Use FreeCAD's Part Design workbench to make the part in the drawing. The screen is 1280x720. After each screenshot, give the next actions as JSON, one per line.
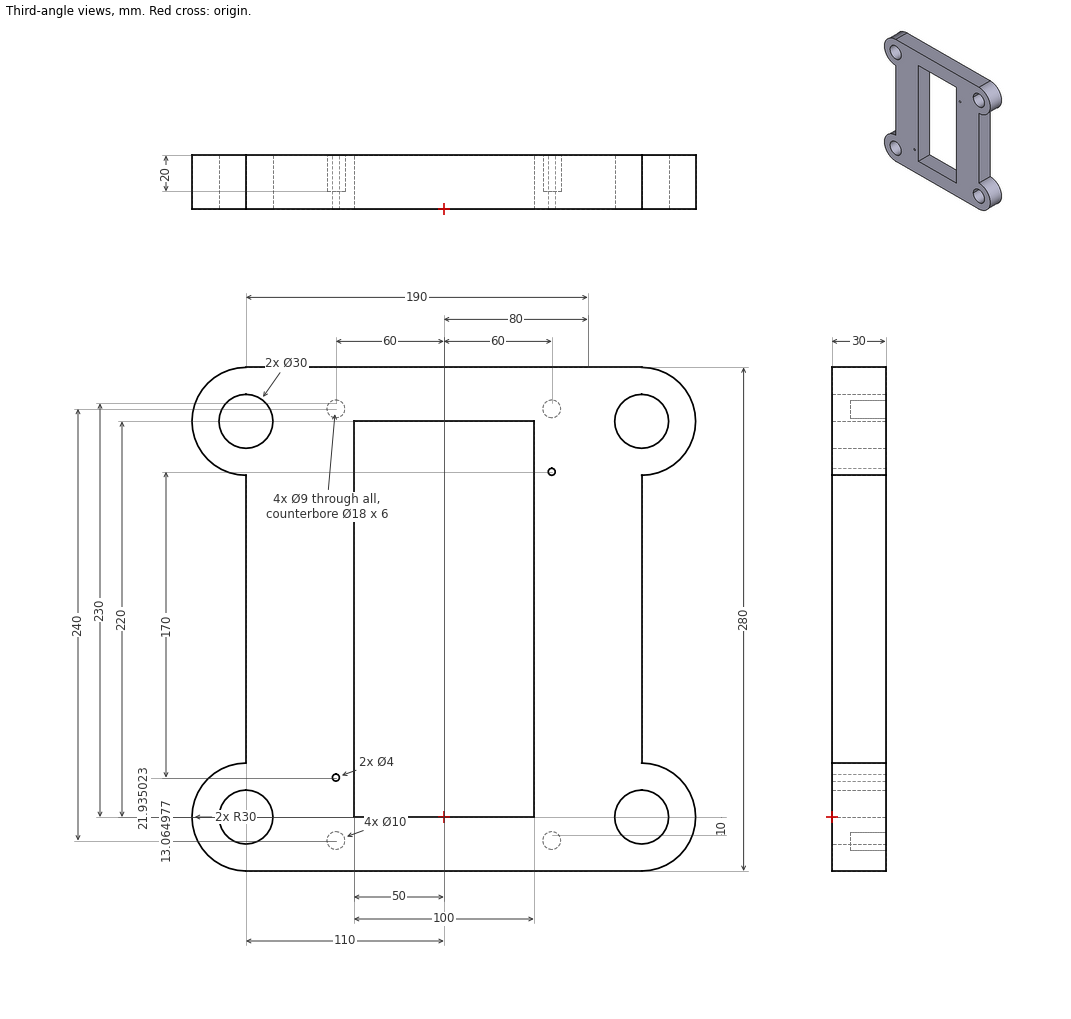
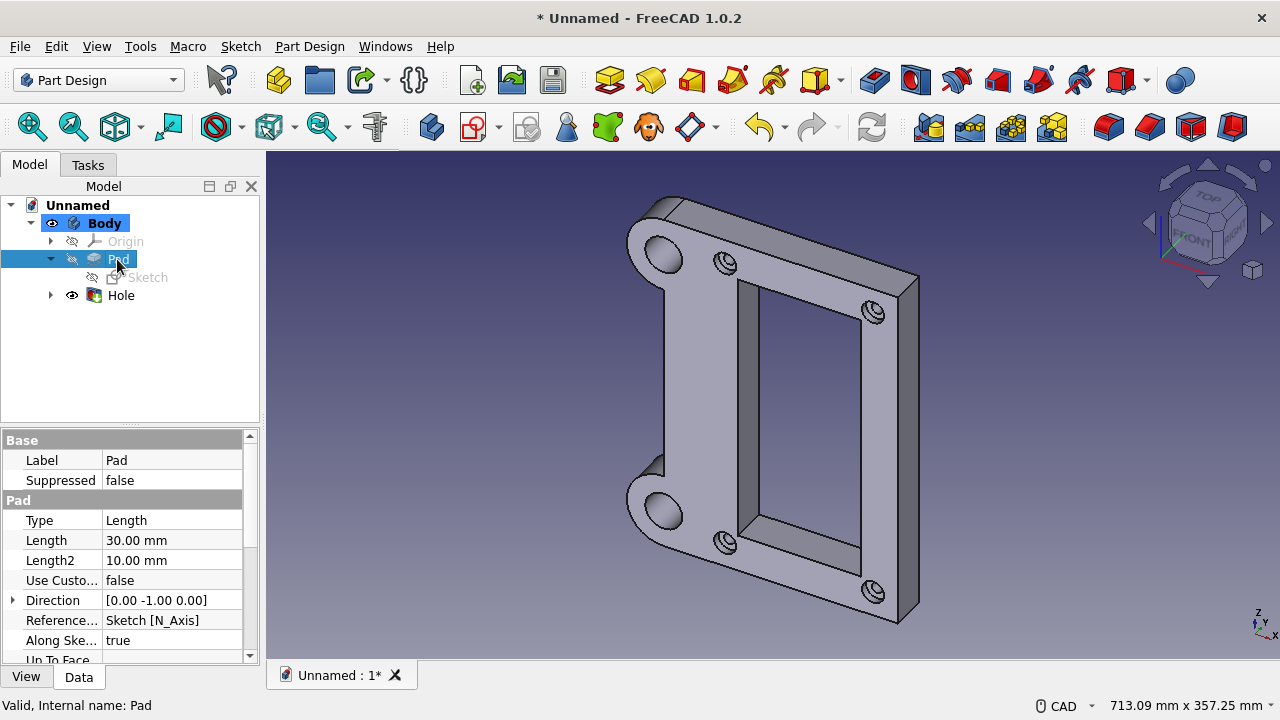
{"action": "left_click", "coordinate": [929, 128]}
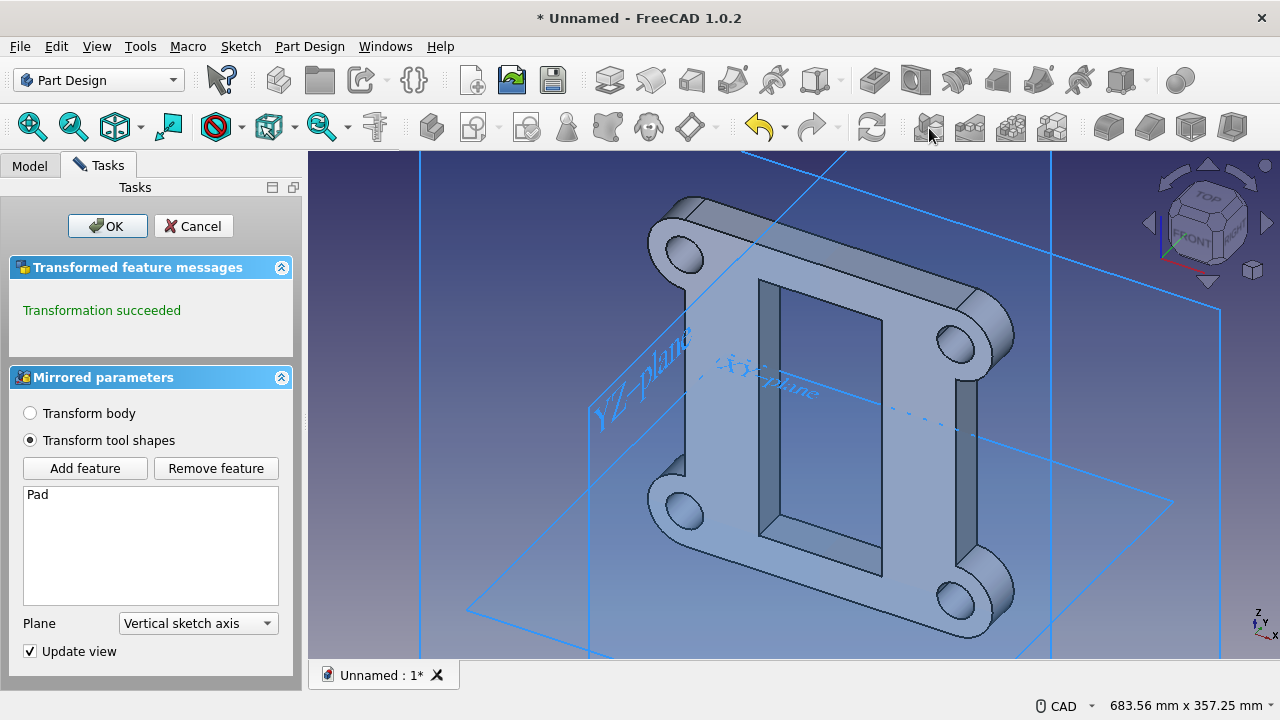
{"action": "left_click", "coordinate": [199, 624]}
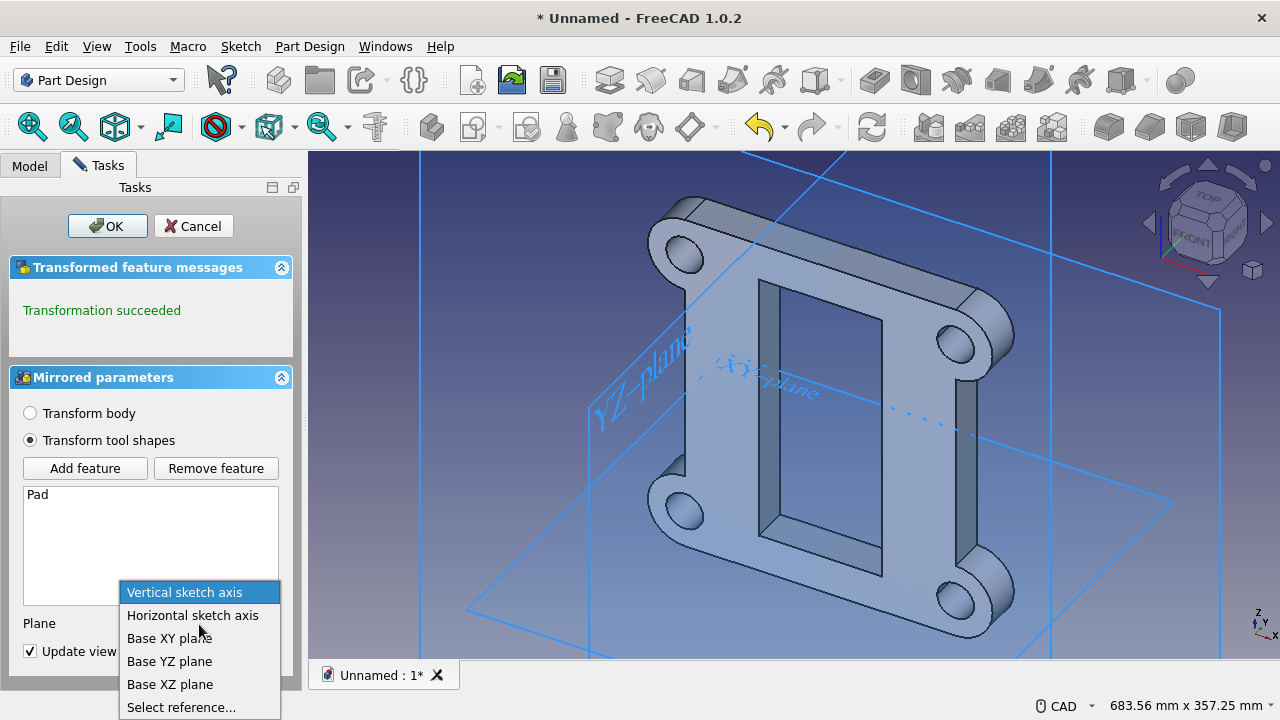
{"action": "left_click", "coordinate": [198, 662]}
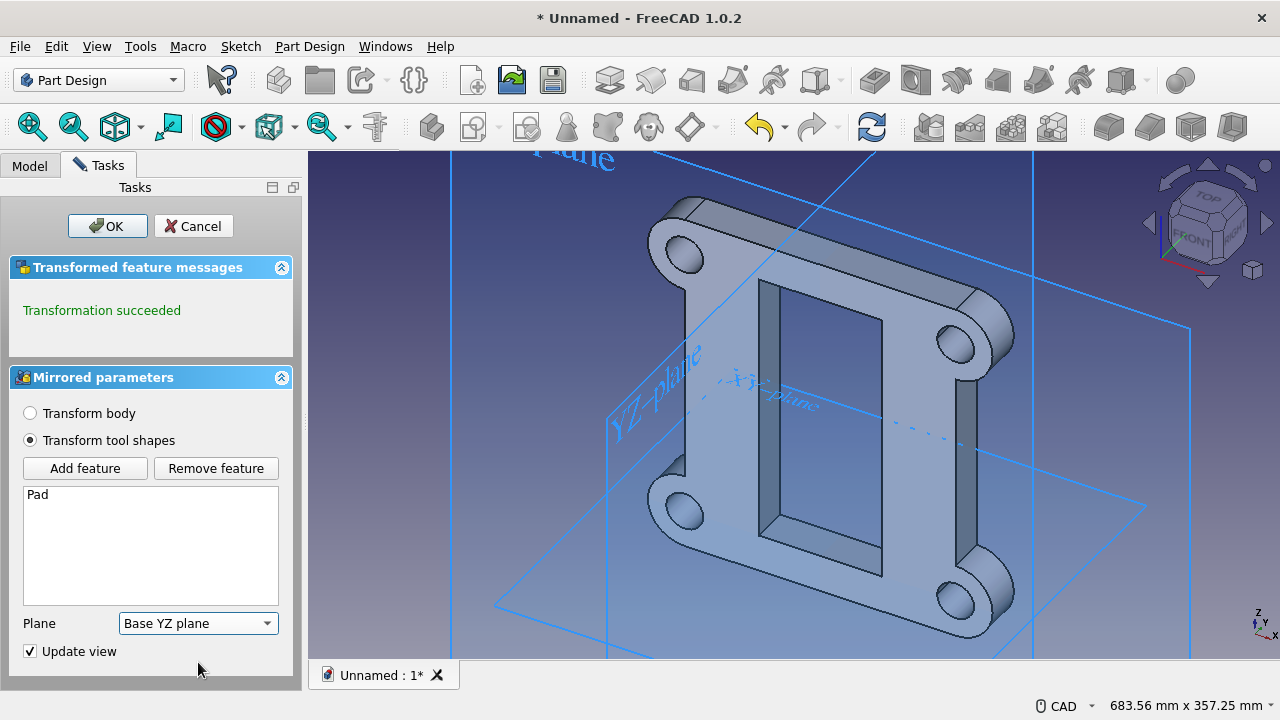
{"action": "left_click", "coordinate": [108, 226]}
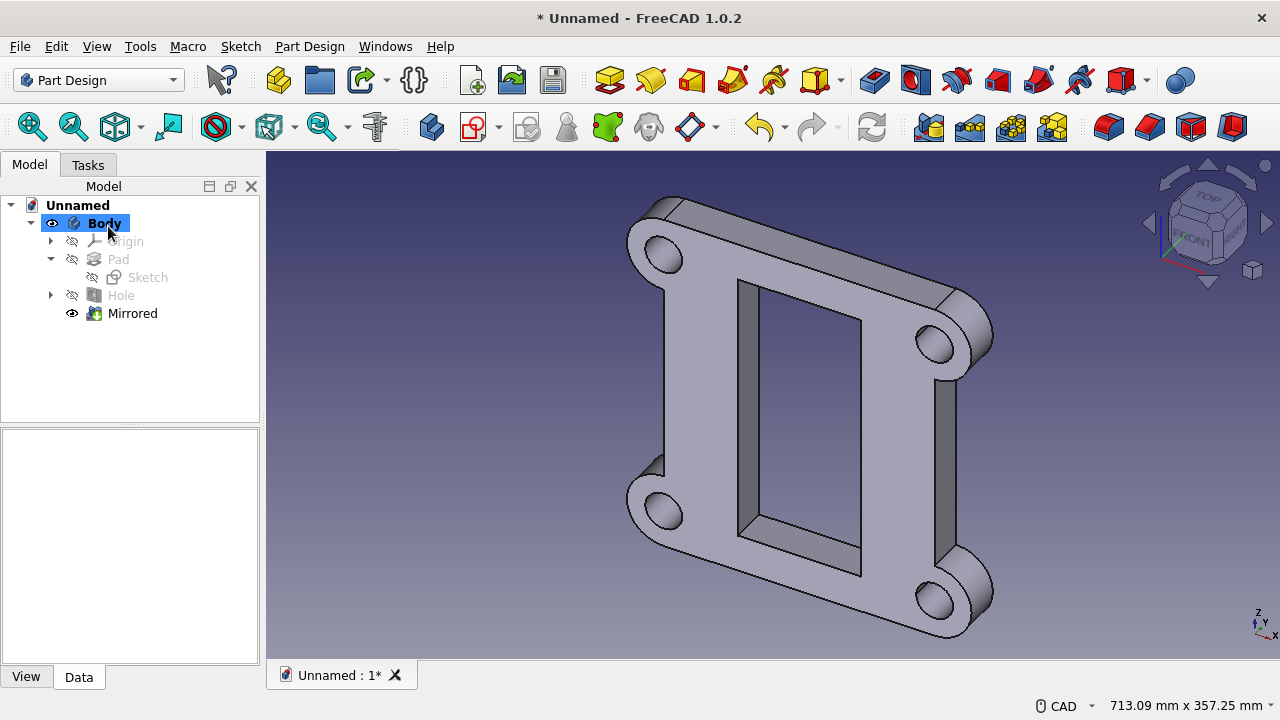
{"action": "key", "text": "4"}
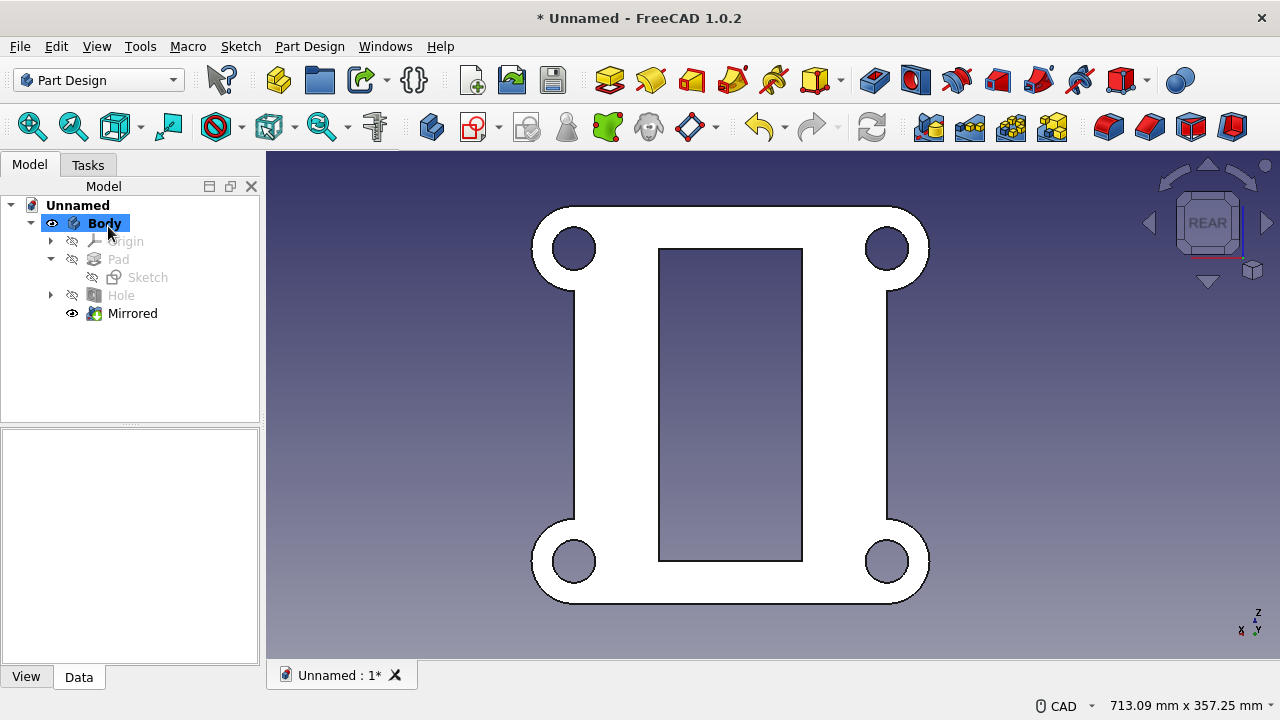
{"action": "left_click", "coordinate": [844, 347]}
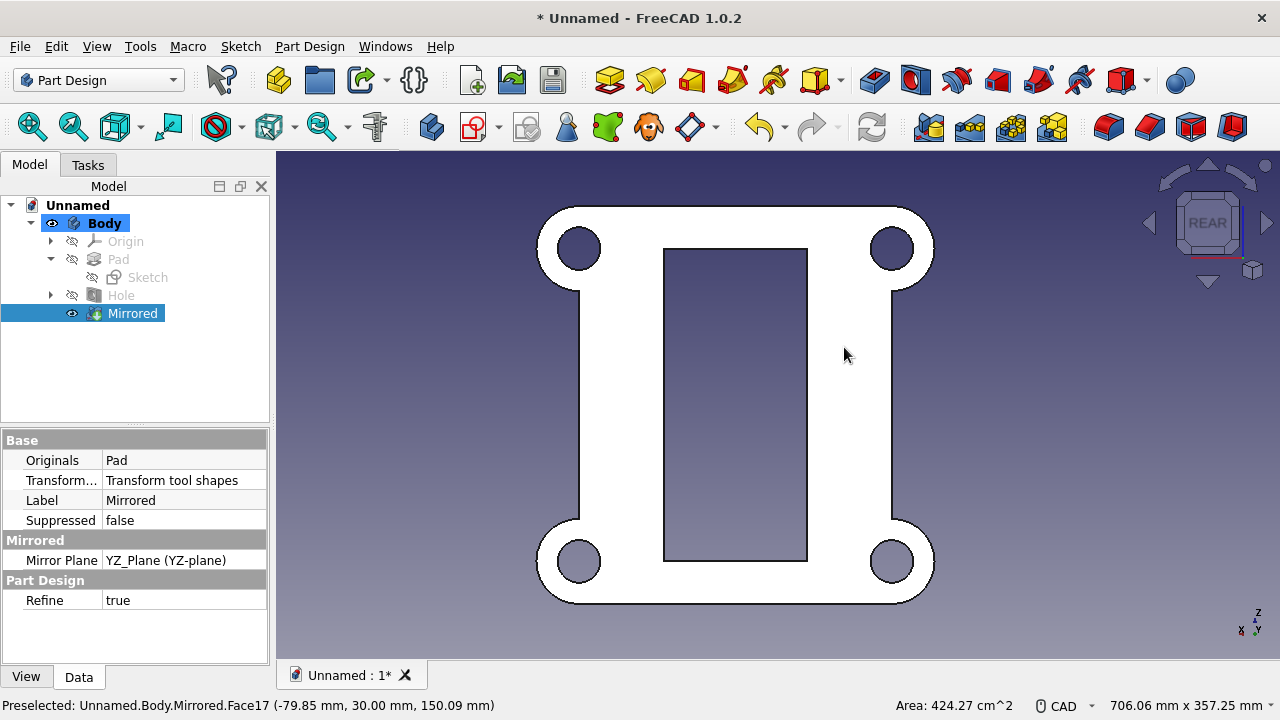
{"action": "left_click", "coordinate": [472, 128]}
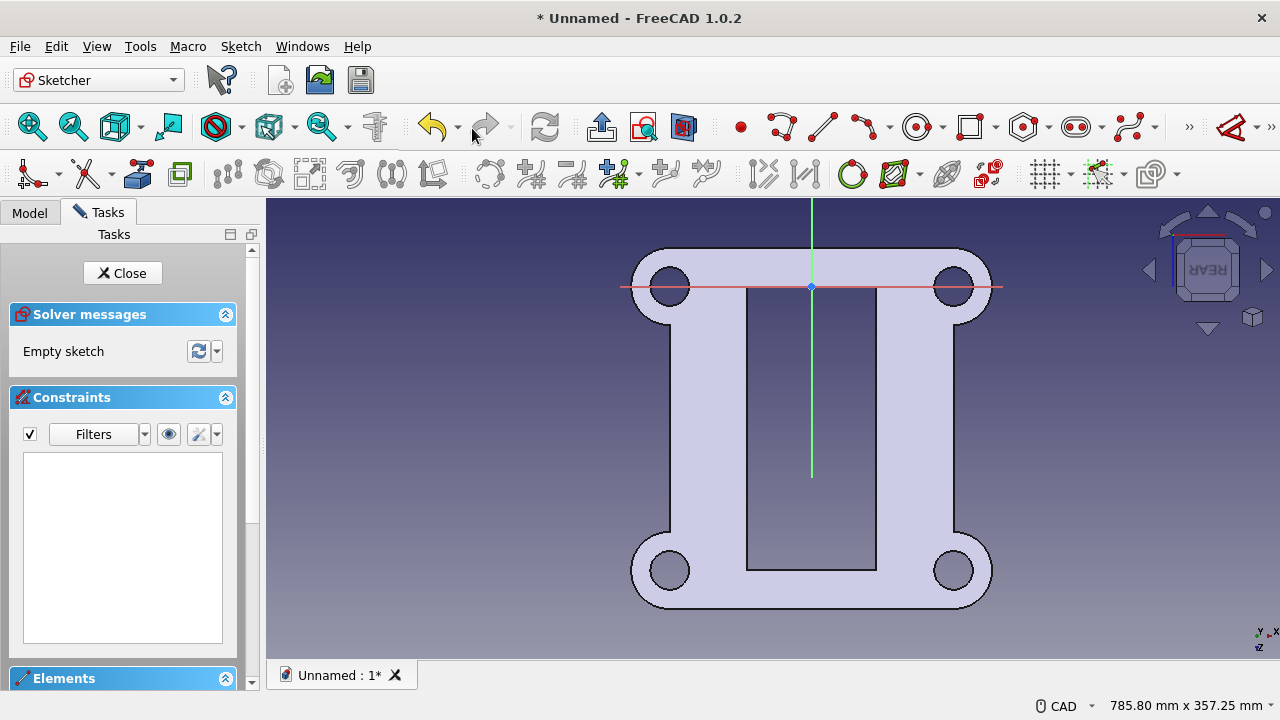
{"action": "key", "text": "g c"}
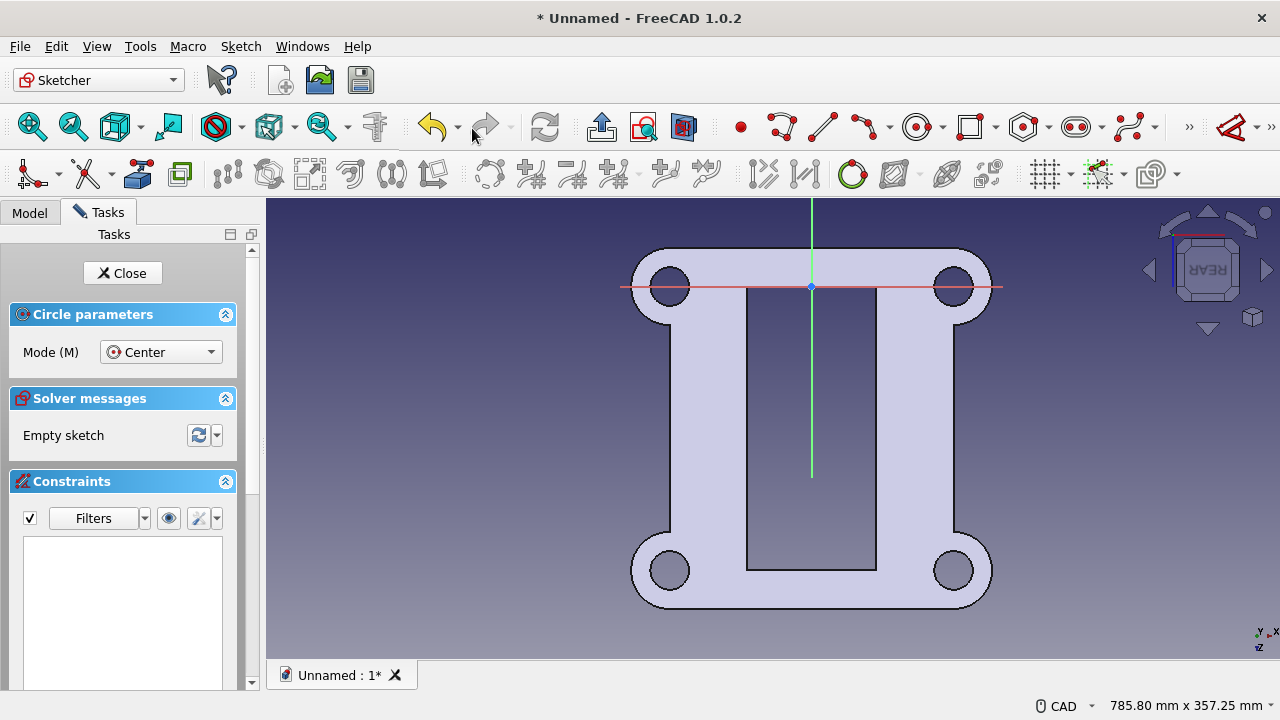
{"action": "scroll", "coordinate": [734, 270], "scroll_direction": "up", "scroll_amount": 7}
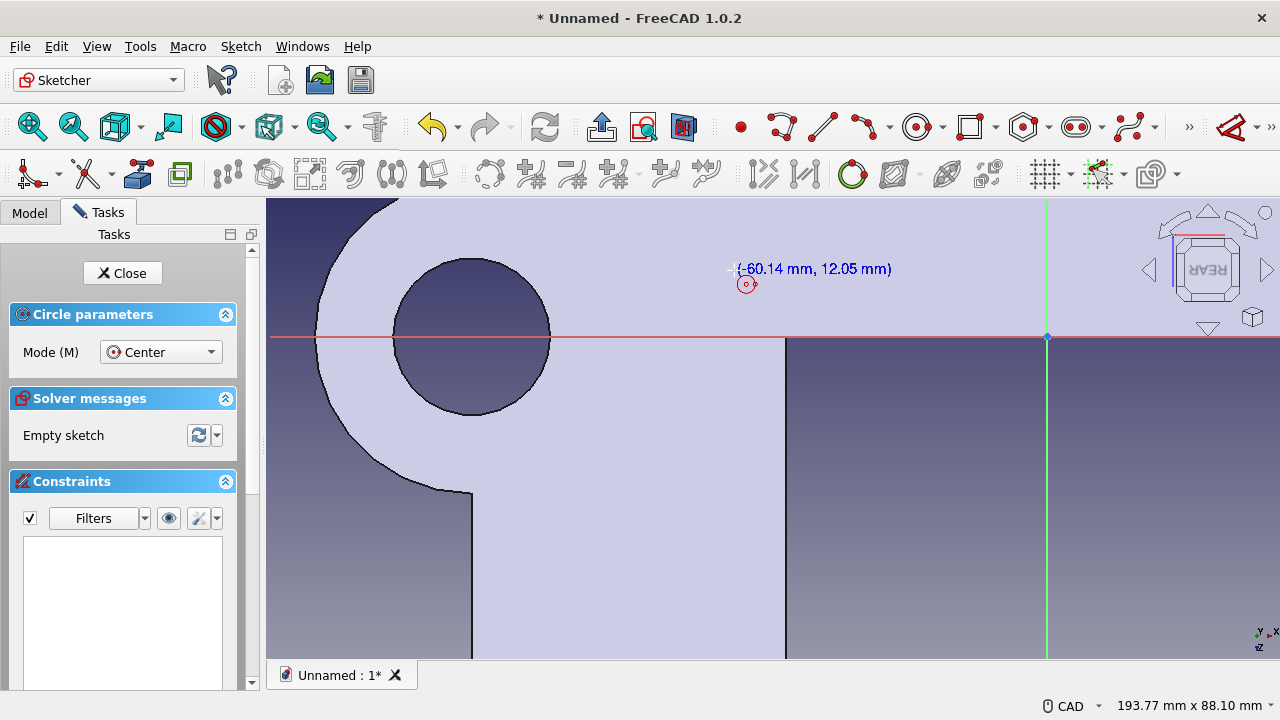
{"action": "scroll", "coordinate": [618, 310], "scroll_direction": "down", "scroll_amount": 8}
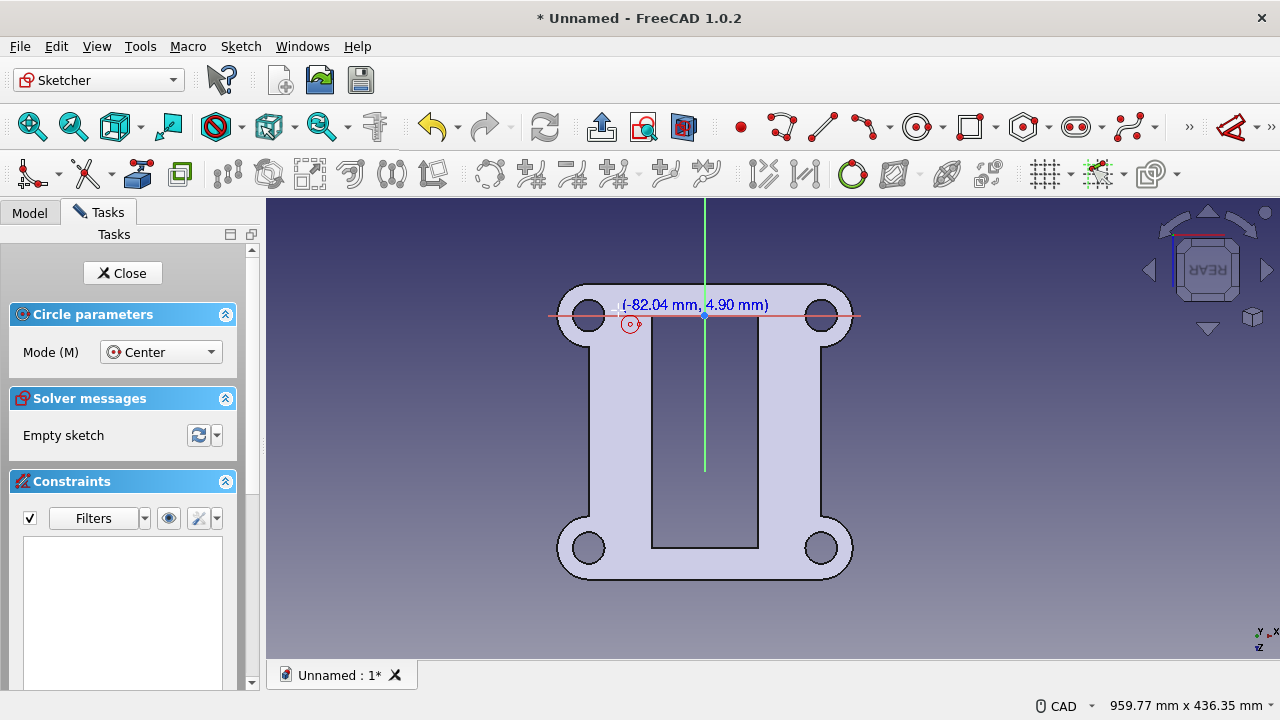
{"action": "left_click", "coordinate": [642, 302]}